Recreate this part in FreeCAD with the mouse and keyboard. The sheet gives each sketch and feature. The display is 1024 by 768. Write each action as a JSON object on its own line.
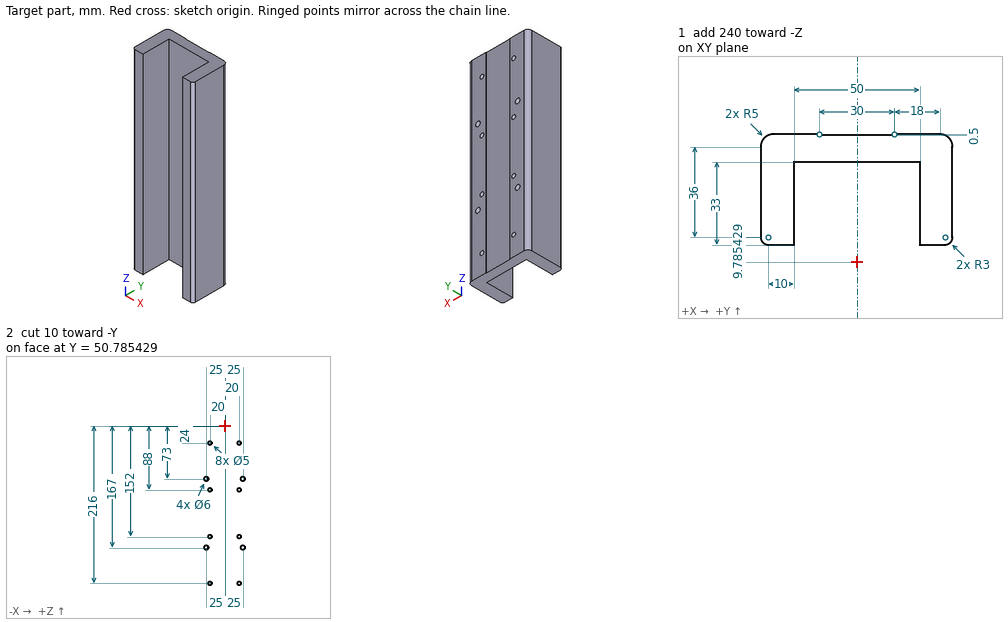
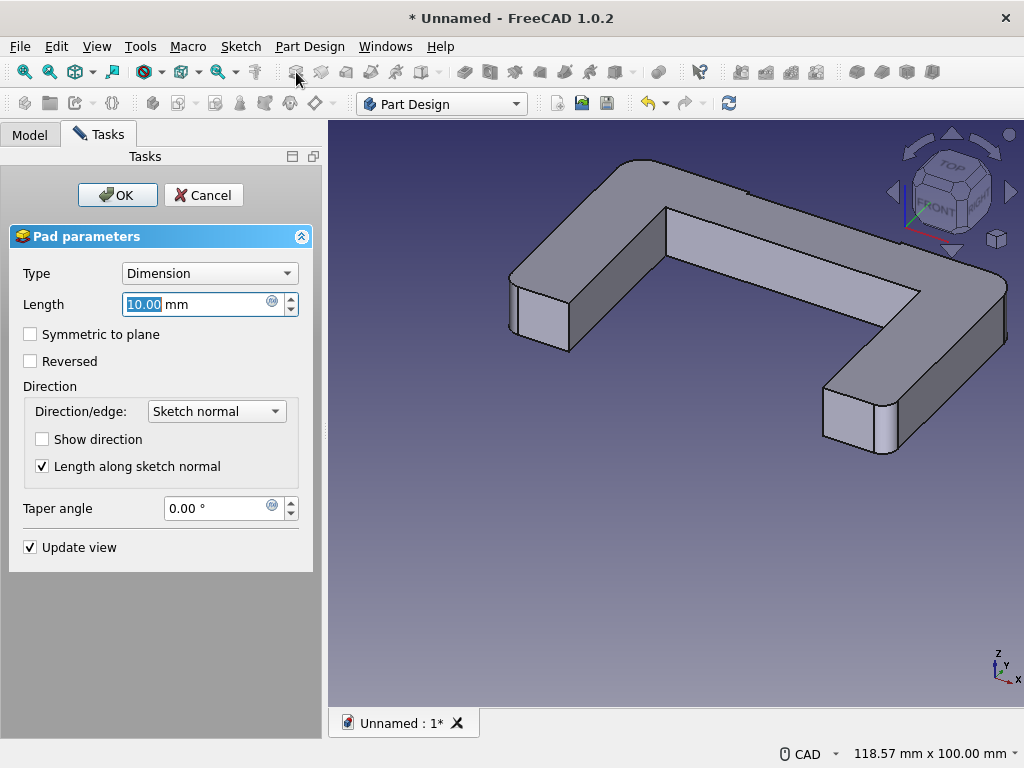
{"action": "type", "text": "240"}
{"action": "key", "text": "Tab"}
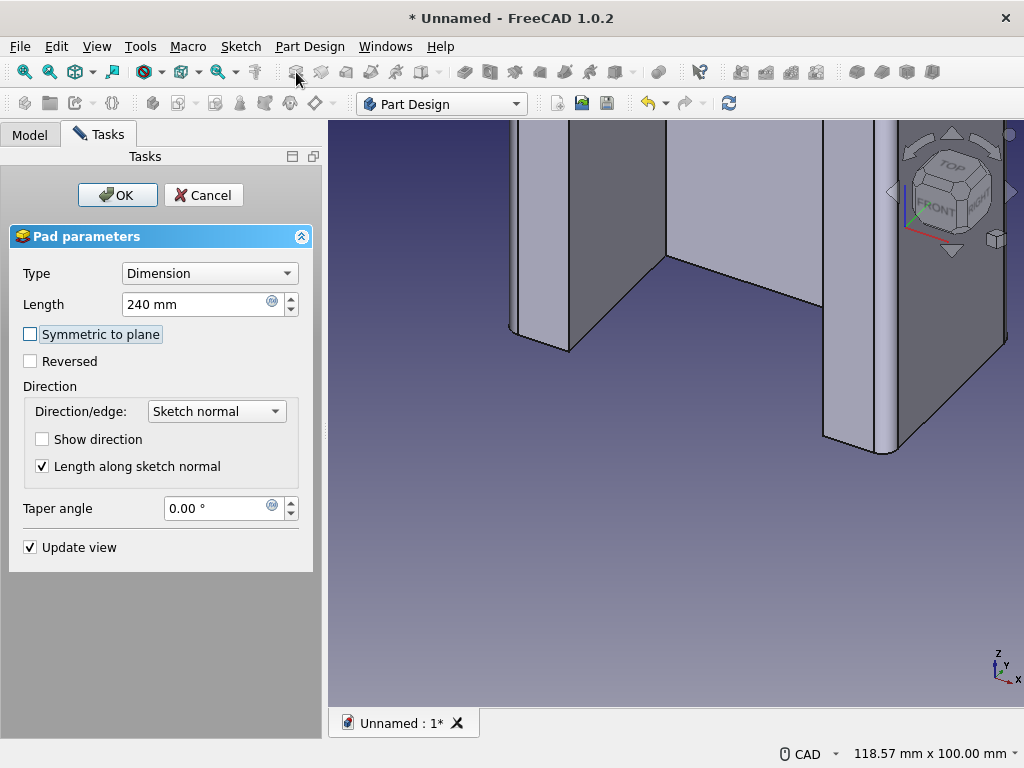
{"action": "left_click", "coordinate": [31, 361]}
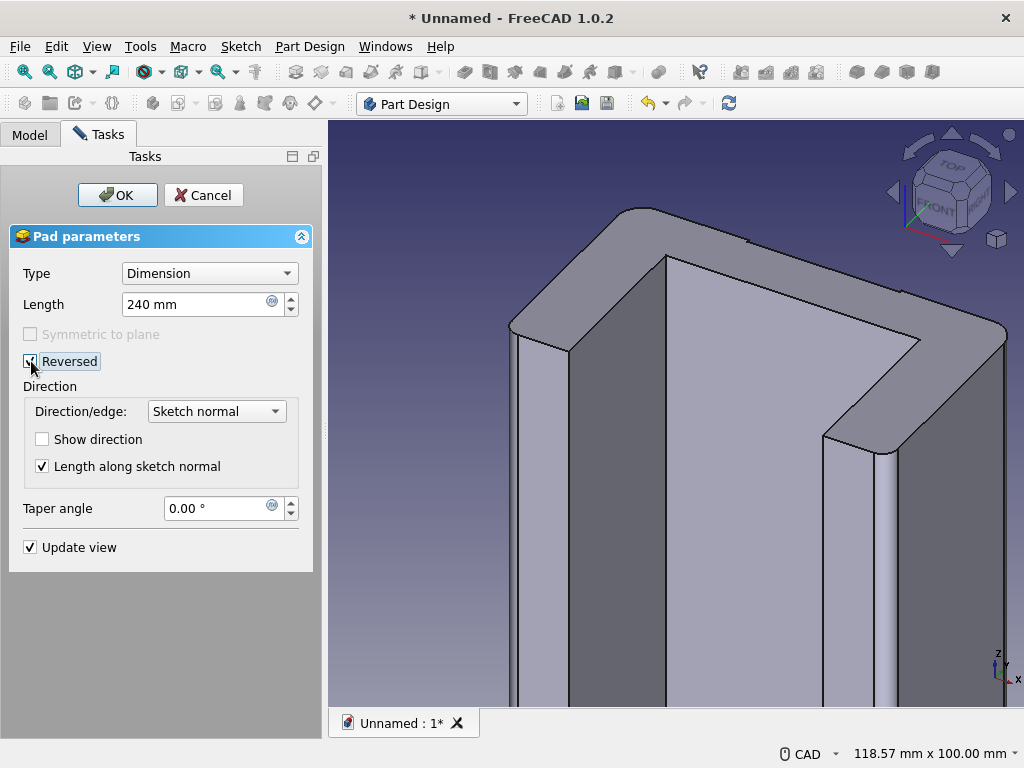
{"action": "left_click", "coordinate": [118, 195]}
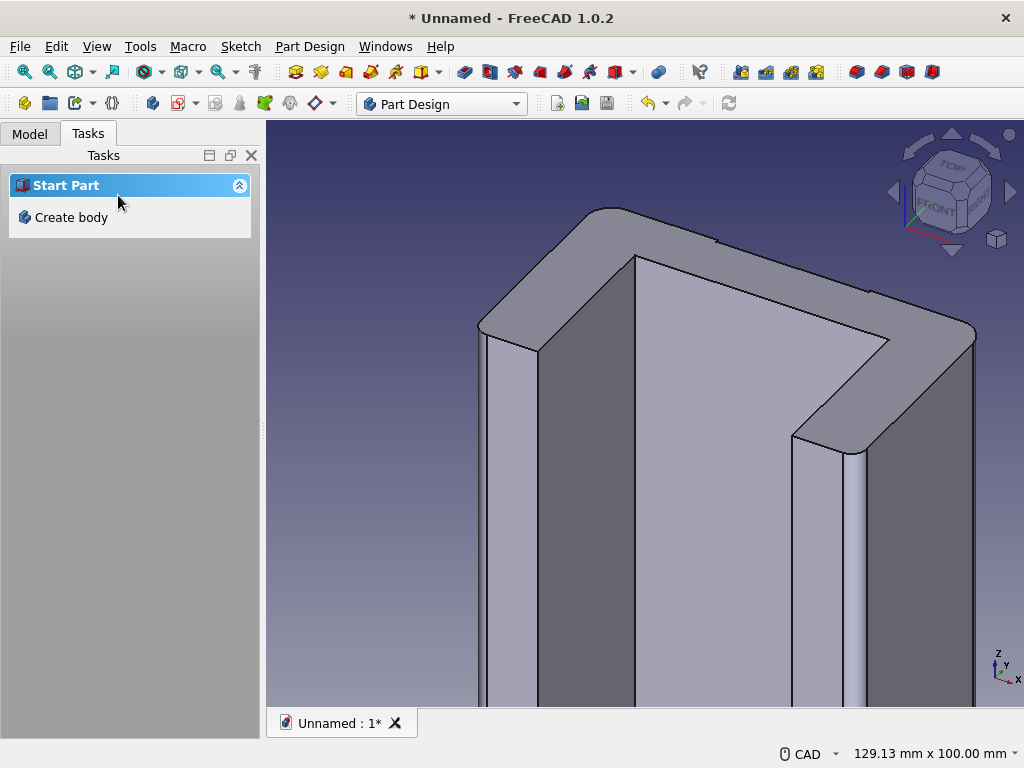
{"action": "left_click", "coordinate": [25, 72]}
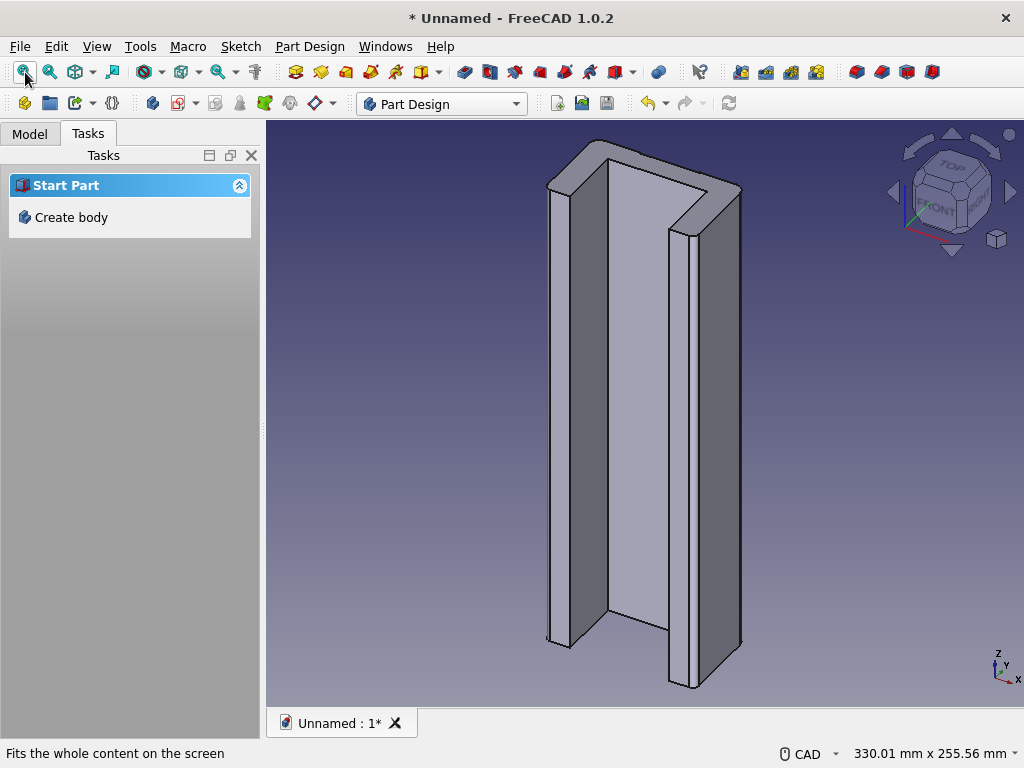
{"action": "key", "text": "4"}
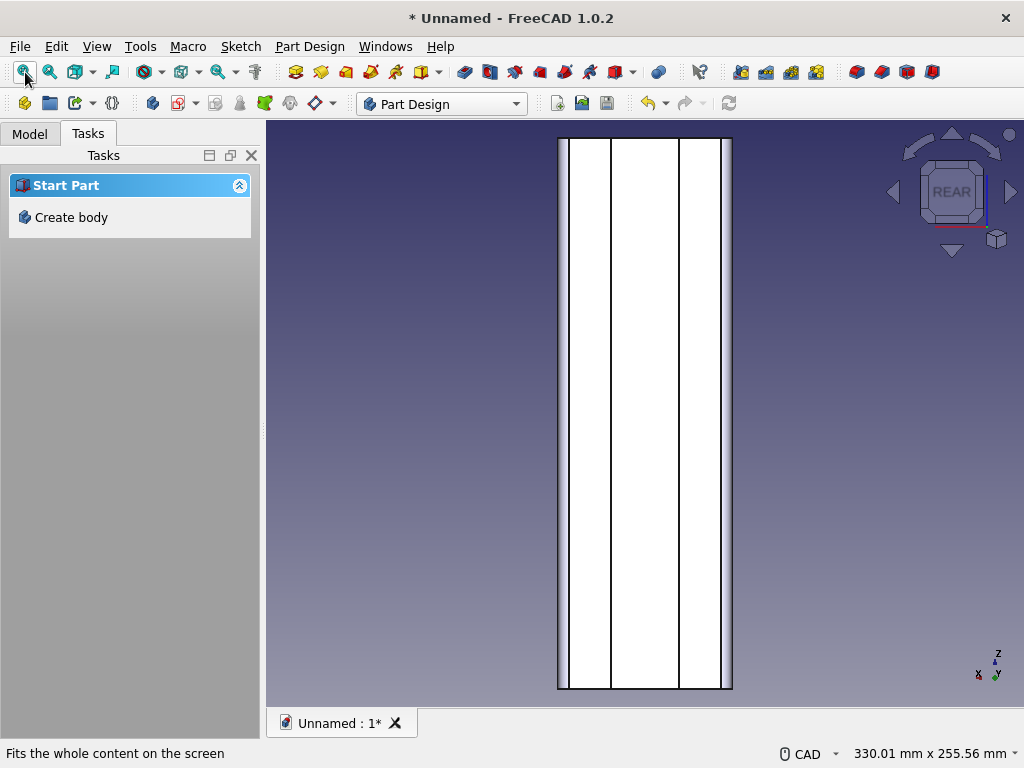
{"action": "left_click", "coordinate": [700, 176]}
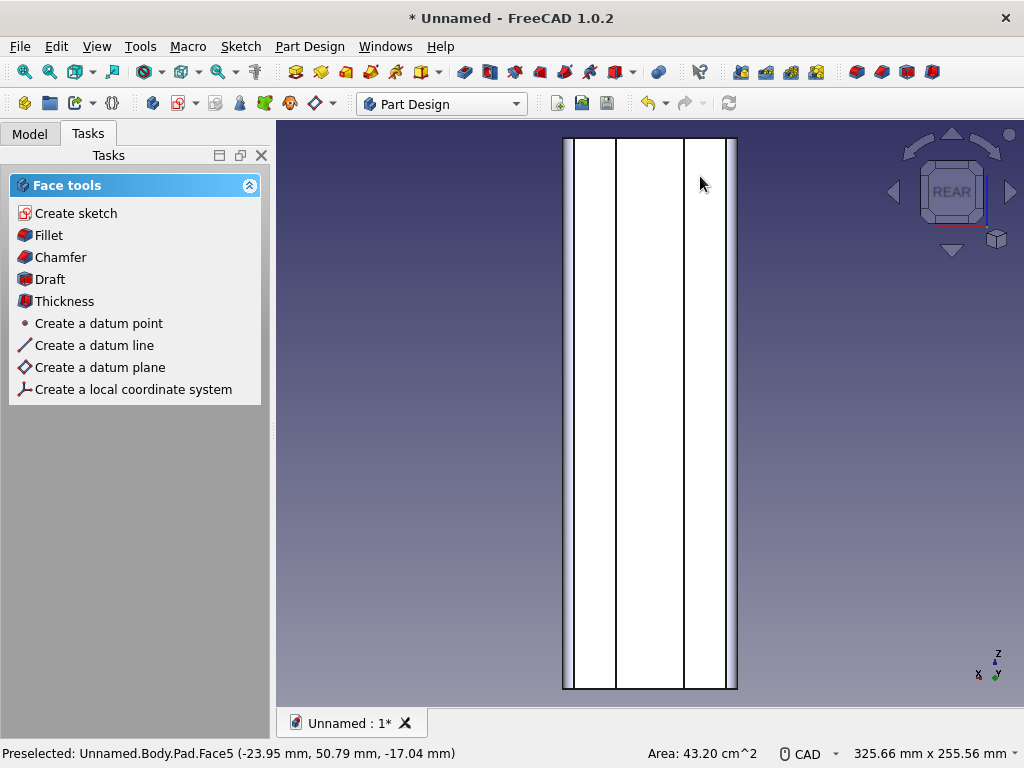
{"action": "left_click", "coordinate": [178, 104]}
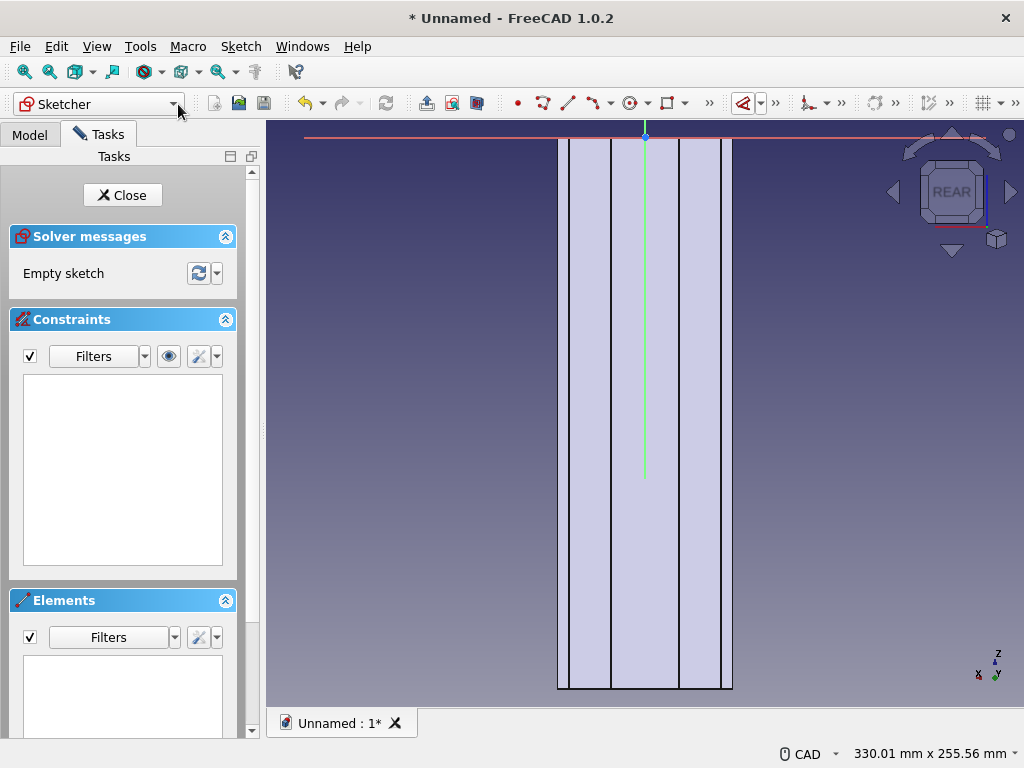
{"action": "scroll", "coordinate": [294, 525], "scroll_direction": "down", "scroll_amount": 1}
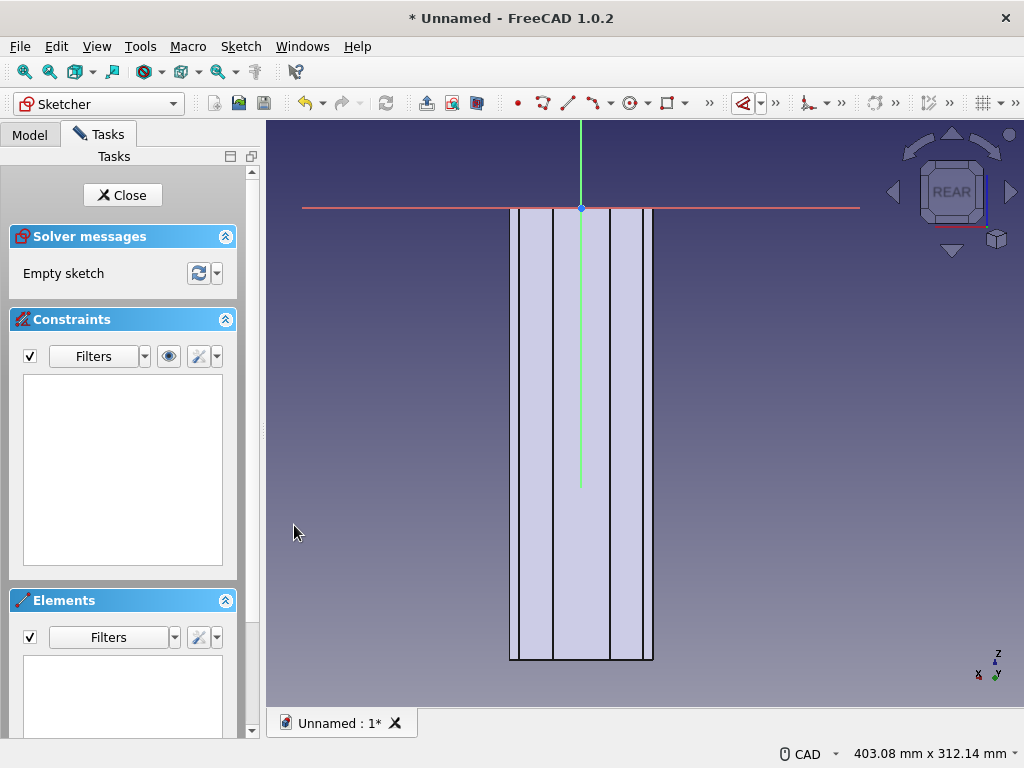
{"action": "left_click", "coordinate": [630, 104]}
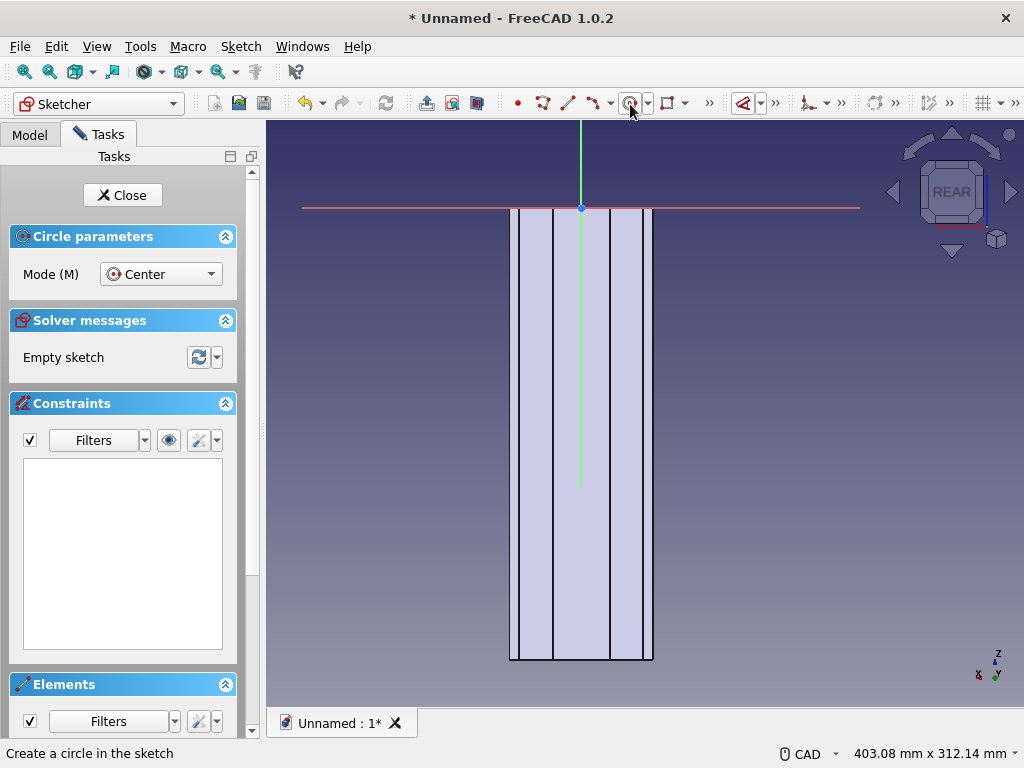
{"action": "scroll", "coordinate": [544, 253], "scroll_direction": "up", "scroll_amount": 8}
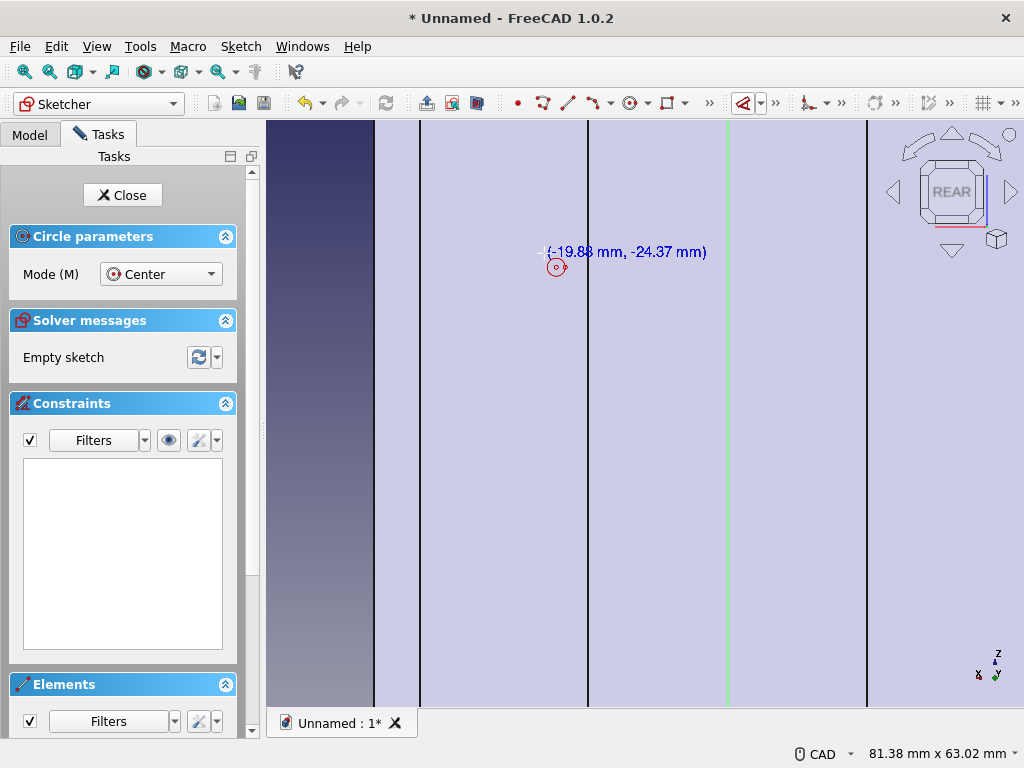
{"action": "scroll", "coordinate": [538, 253], "scroll_direction": "down", "scroll_amount": 8}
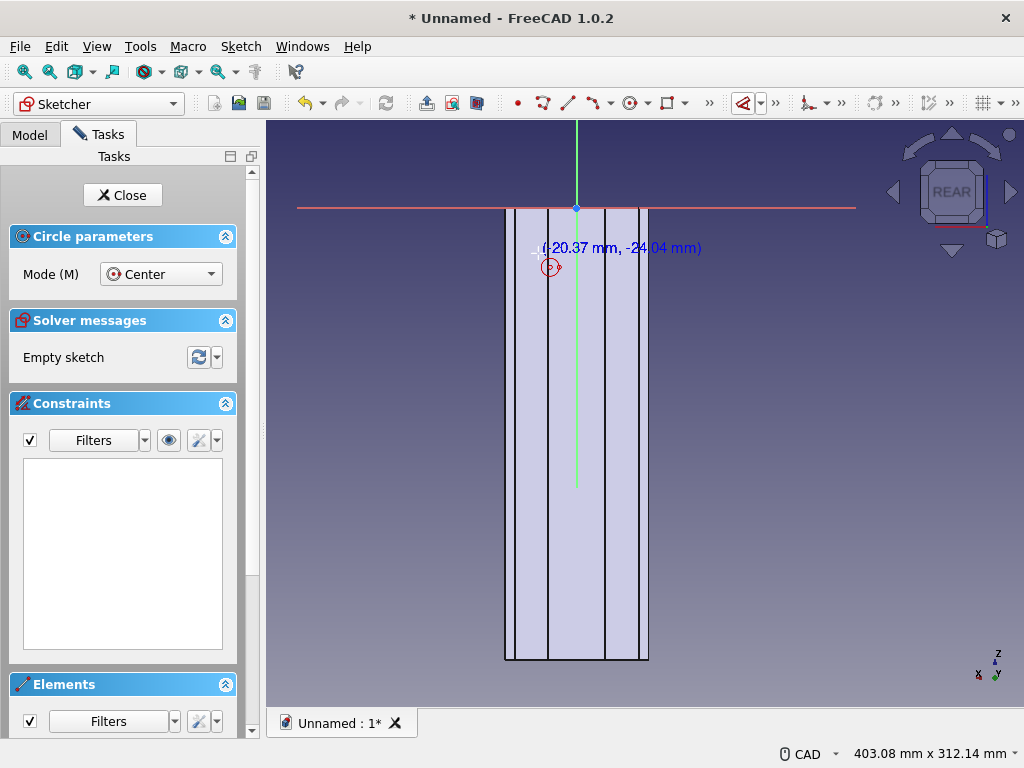
{"action": "left_click", "coordinate": [539, 253]}
{"action": "mouse_move", "coordinate": [542, 250]}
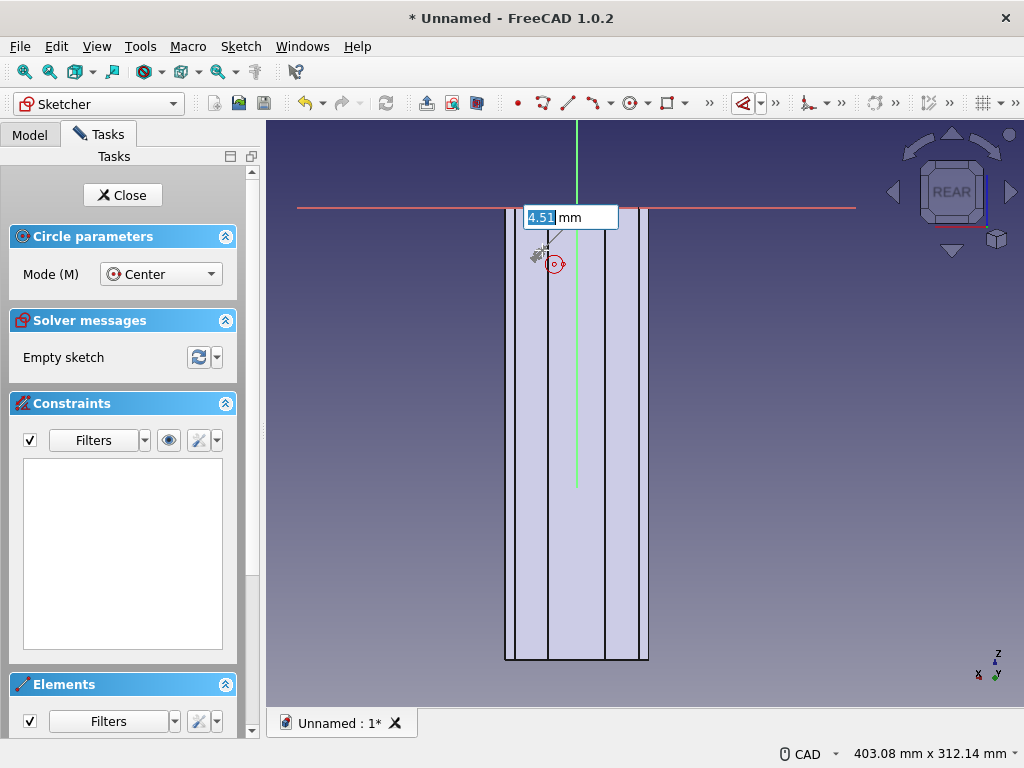
{"action": "type", "text": "5"}
{"action": "key", "text": "Return"}